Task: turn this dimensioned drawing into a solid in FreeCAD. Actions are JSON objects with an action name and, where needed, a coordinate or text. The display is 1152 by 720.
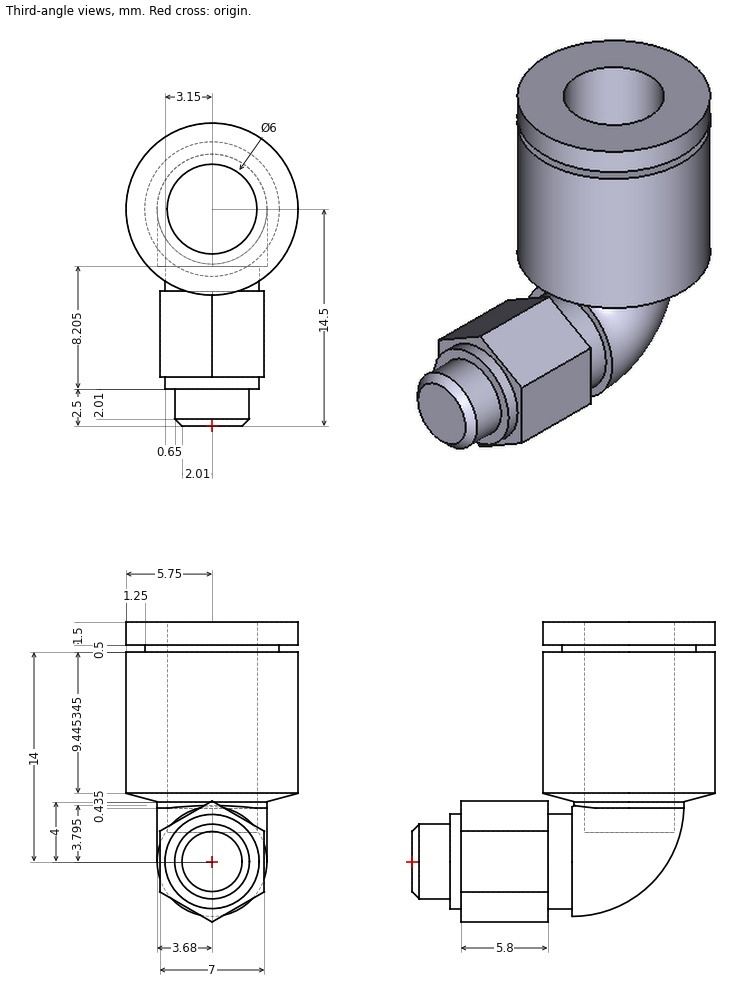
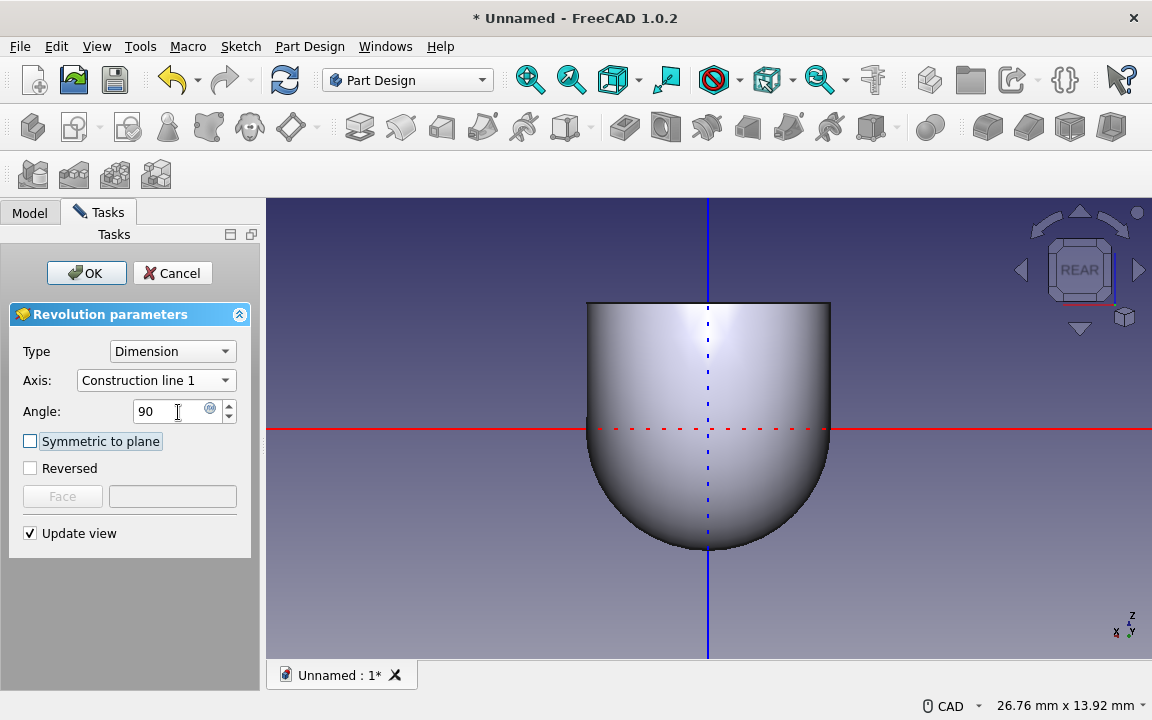
{"action": "left_click", "coordinate": [87, 273]}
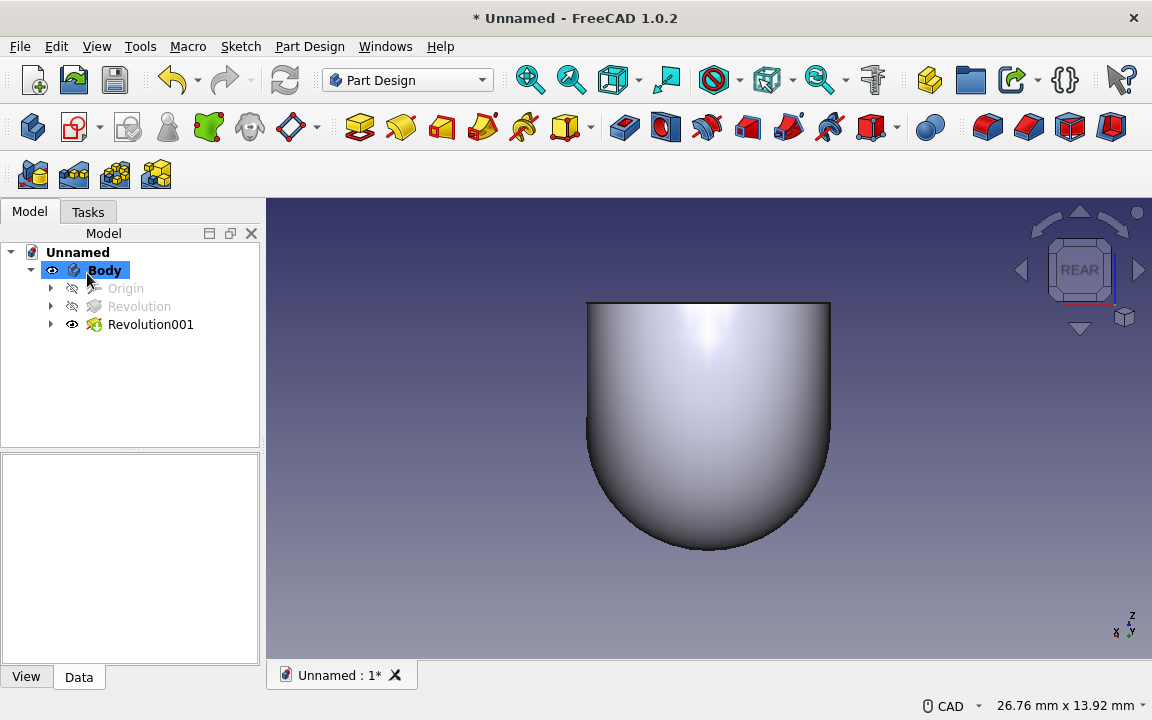
{"action": "left_click", "coordinate": [51, 288]}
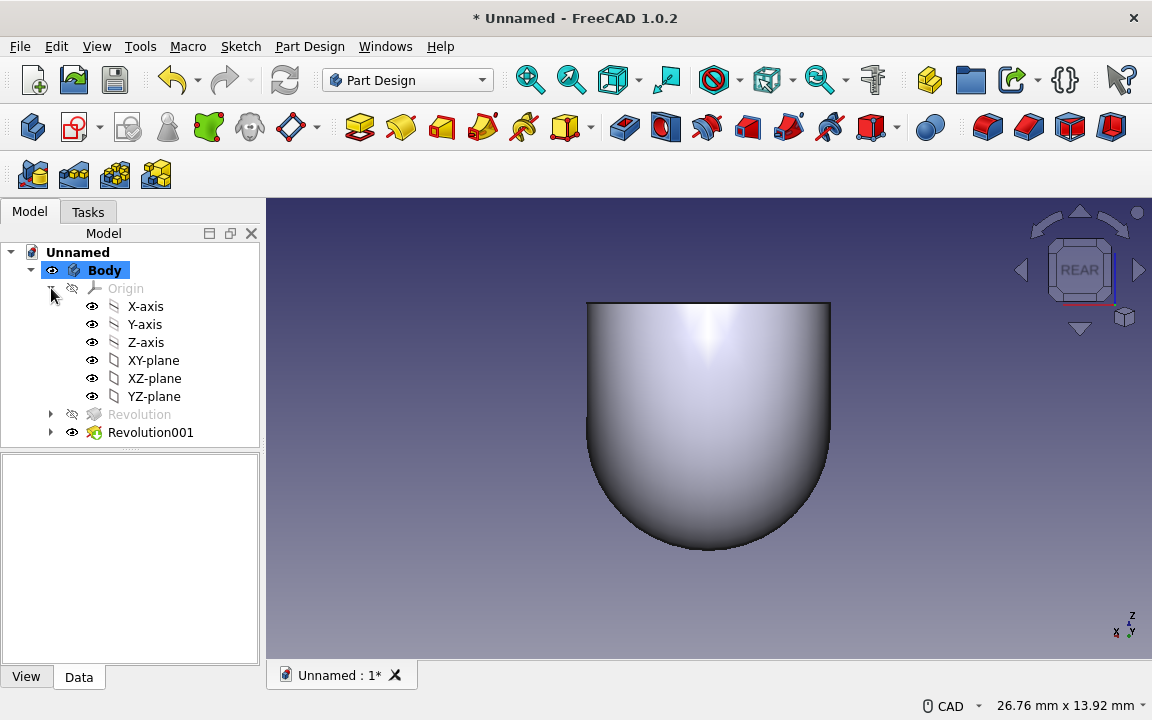
{"action": "left_click", "coordinate": [137, 378]}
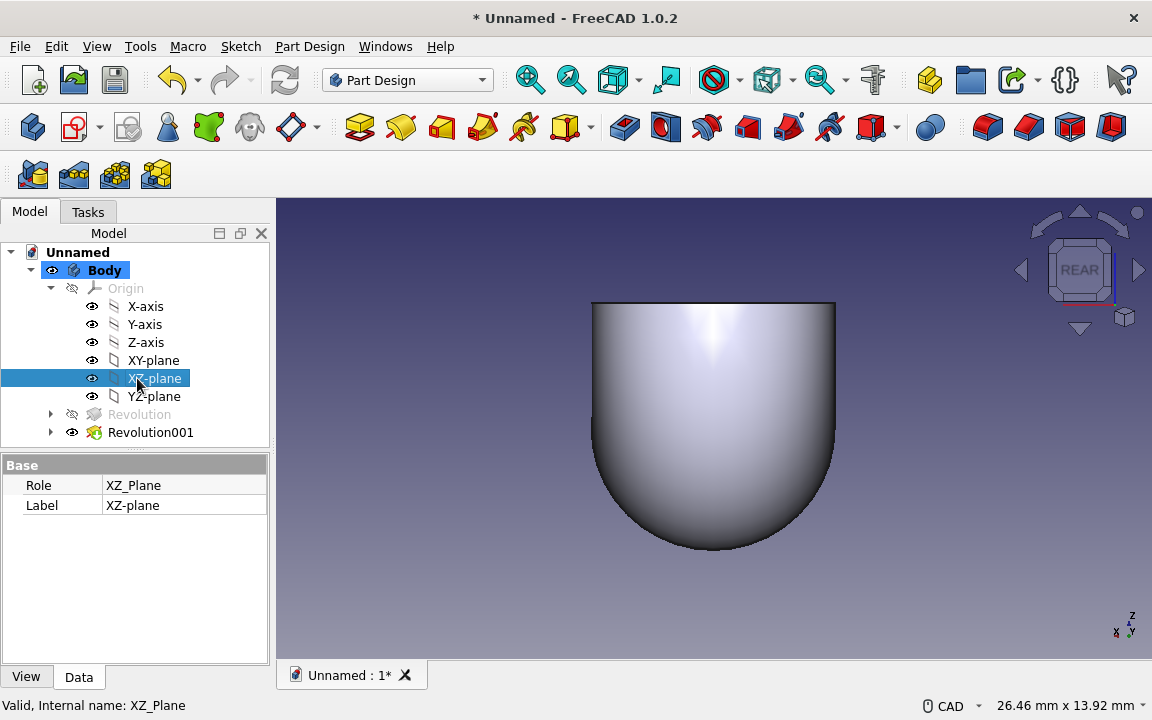
{"action": "left_click", "coordinate": [290, 128]}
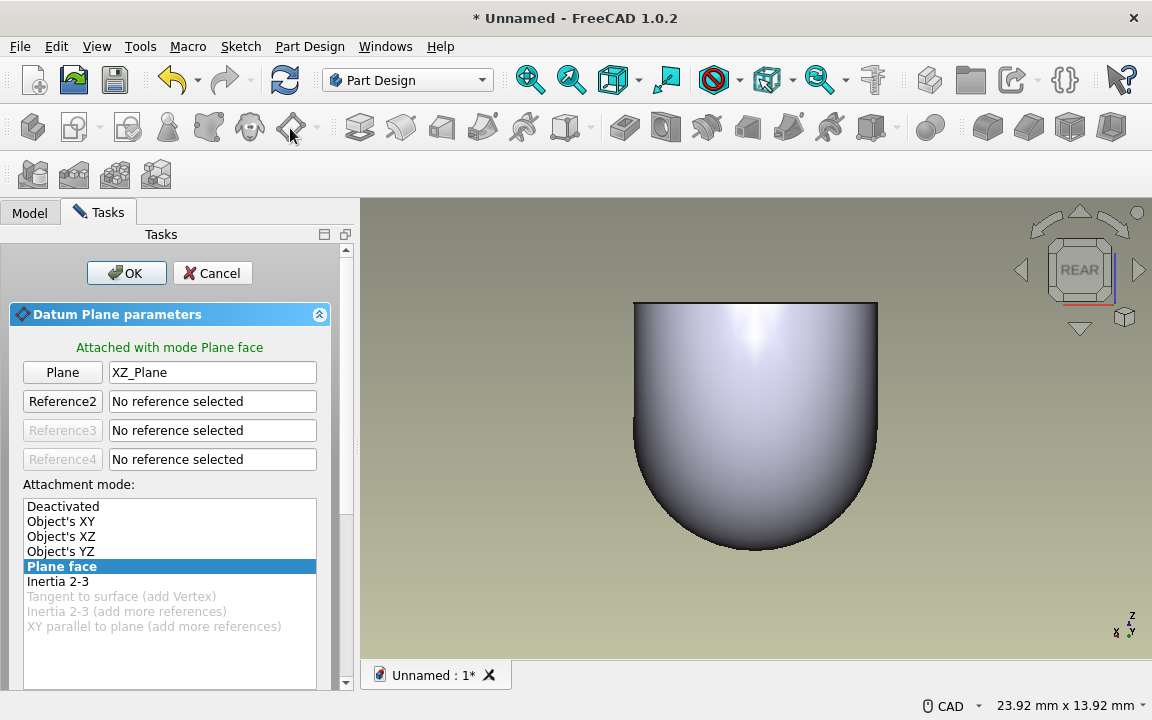
{"action": "scroll", "coordinate": [346, 467], "scroll_direction": "down", "scroll_amount": 4}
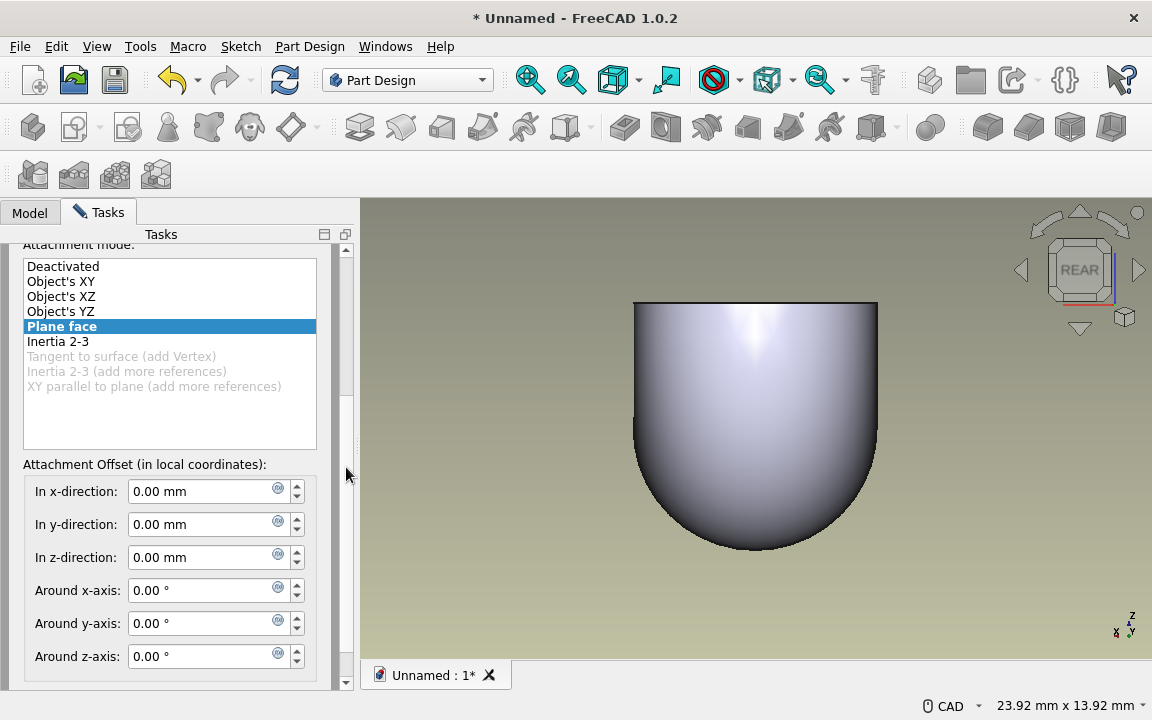
{"action": "triple_click", "coordinate": [210, 558]}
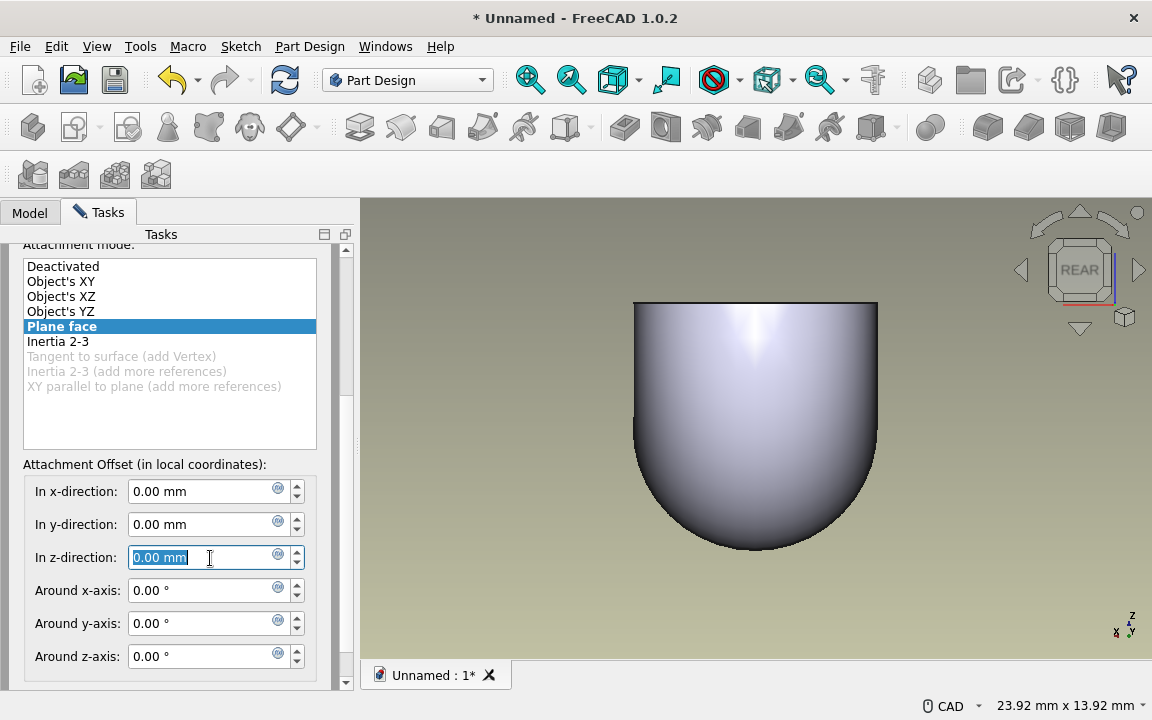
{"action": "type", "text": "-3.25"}
{"action": "key", "text": "Tab"}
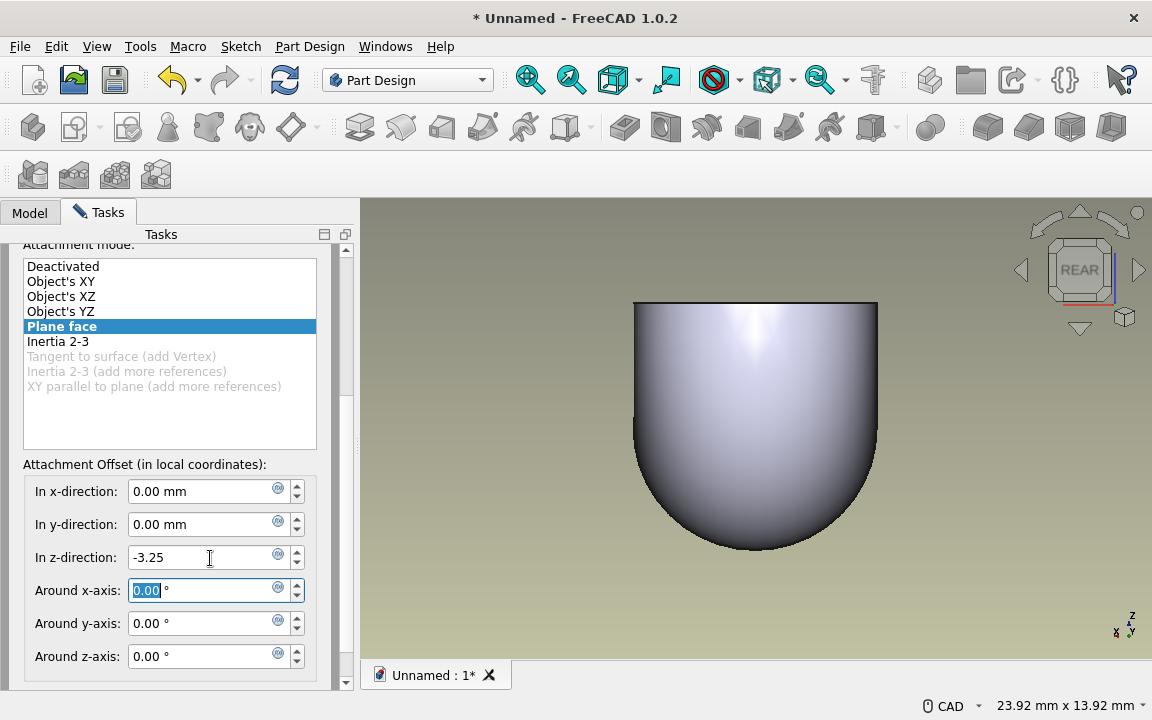
{"action": "scroll", "coordinate": [346, 467], "scroll_direction": "up", "scroll_amount": 5}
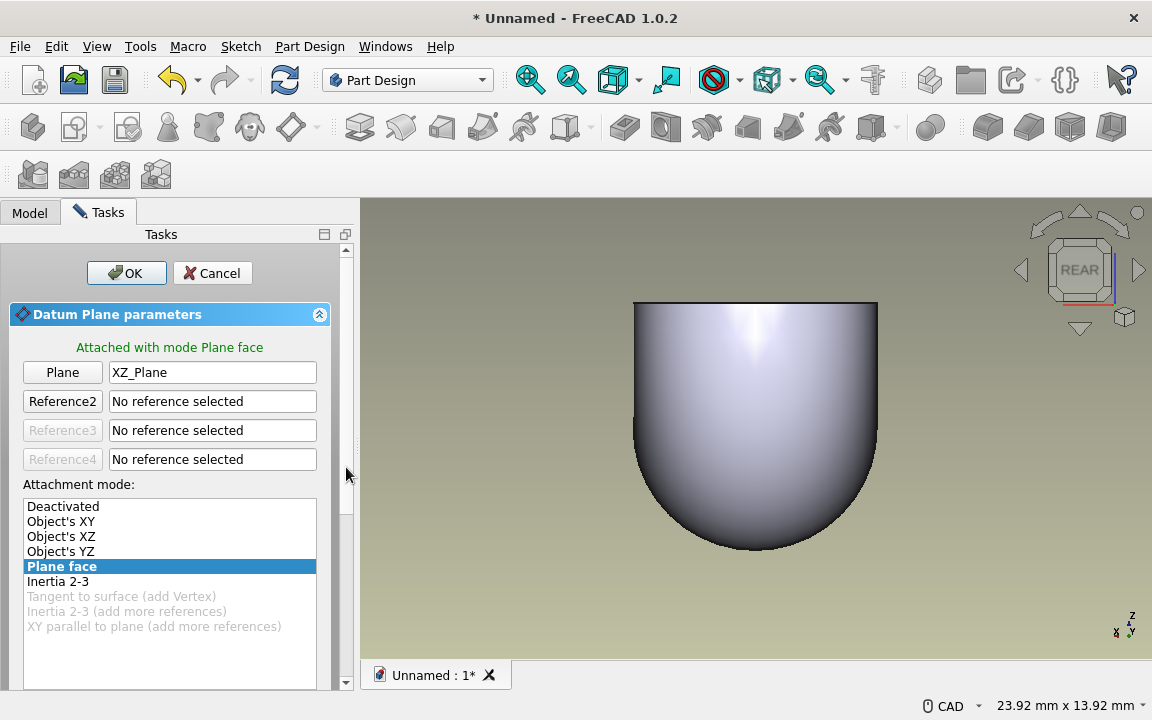
{"action": "left_click", "coordinate": [127, 273]}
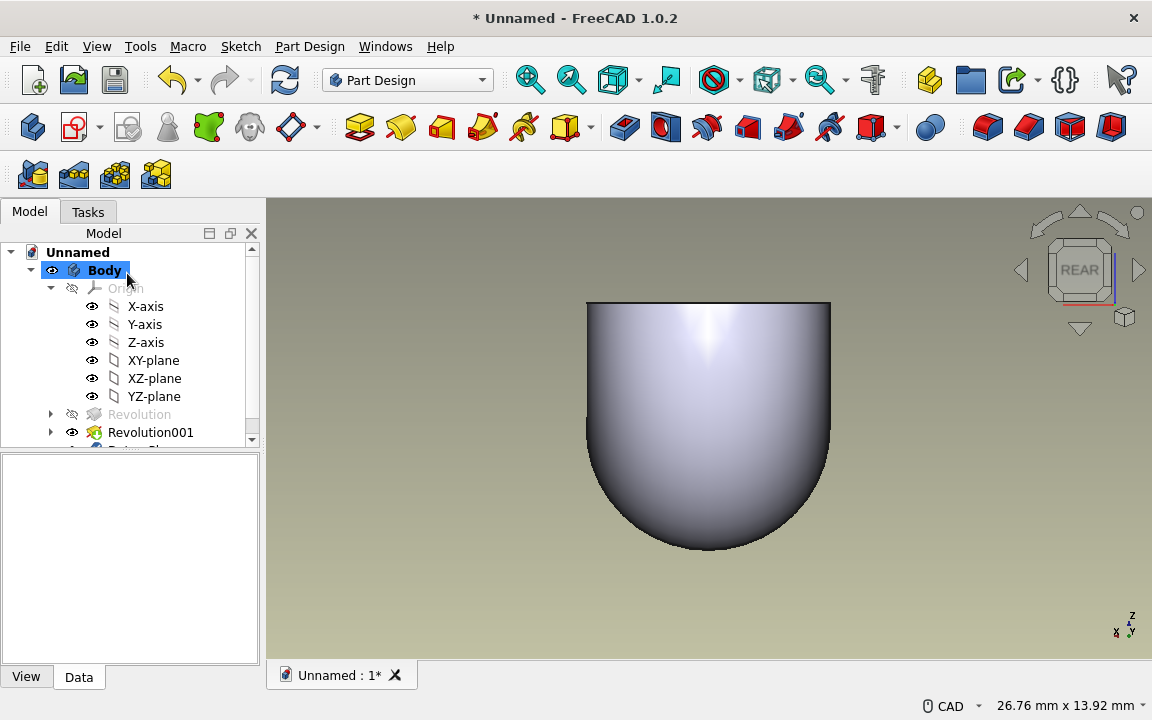
{"action": "scroll", "coordinate": [101, 338], "scroll_direction": "down", "scroll_amount": 3}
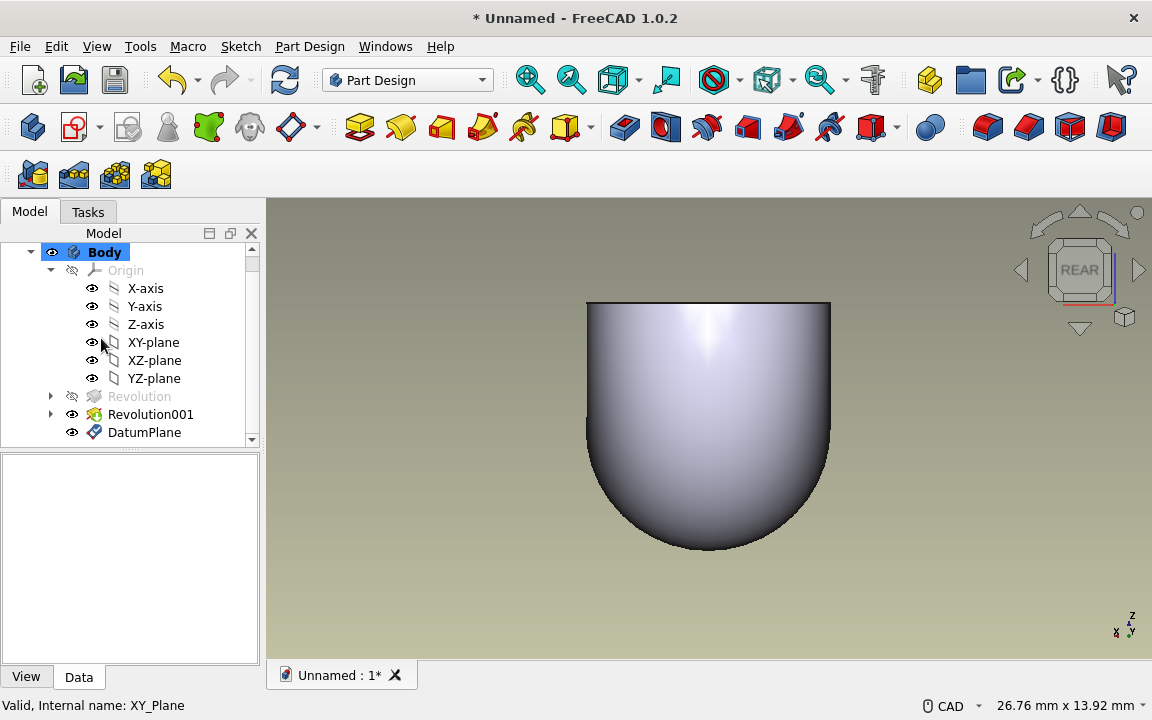
{"action": "left_click", "coordinate": [117, 432]}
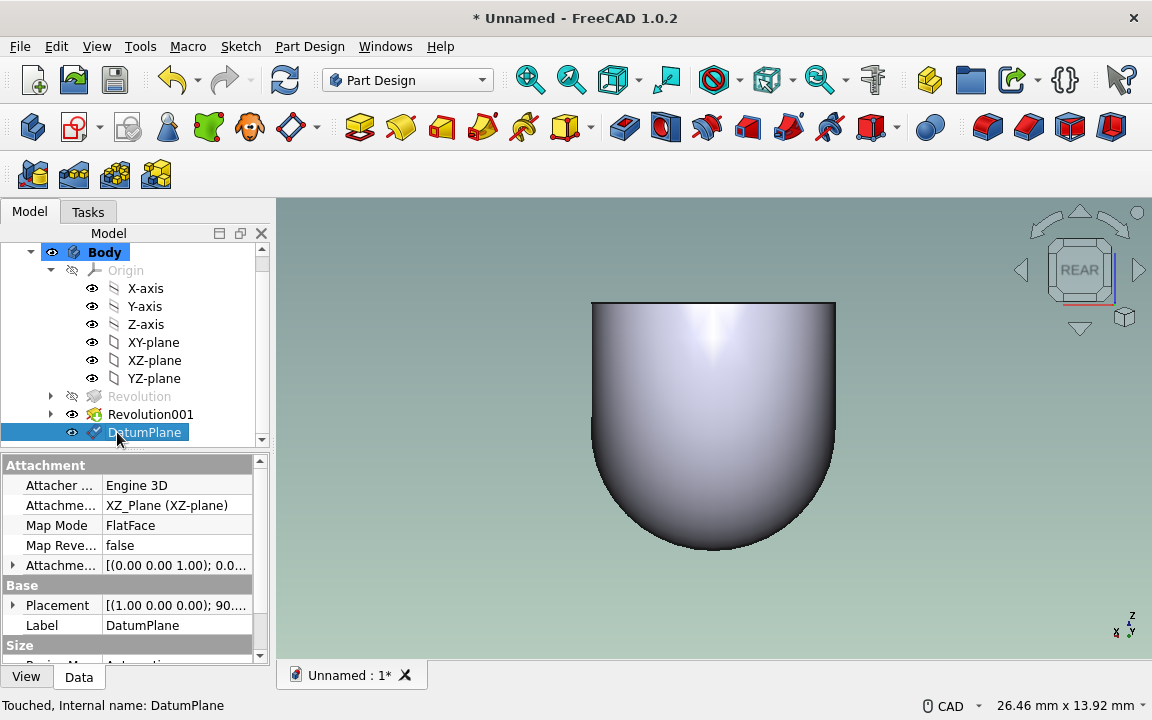
{"action": "left_click", "coordinate": [74, 128]}